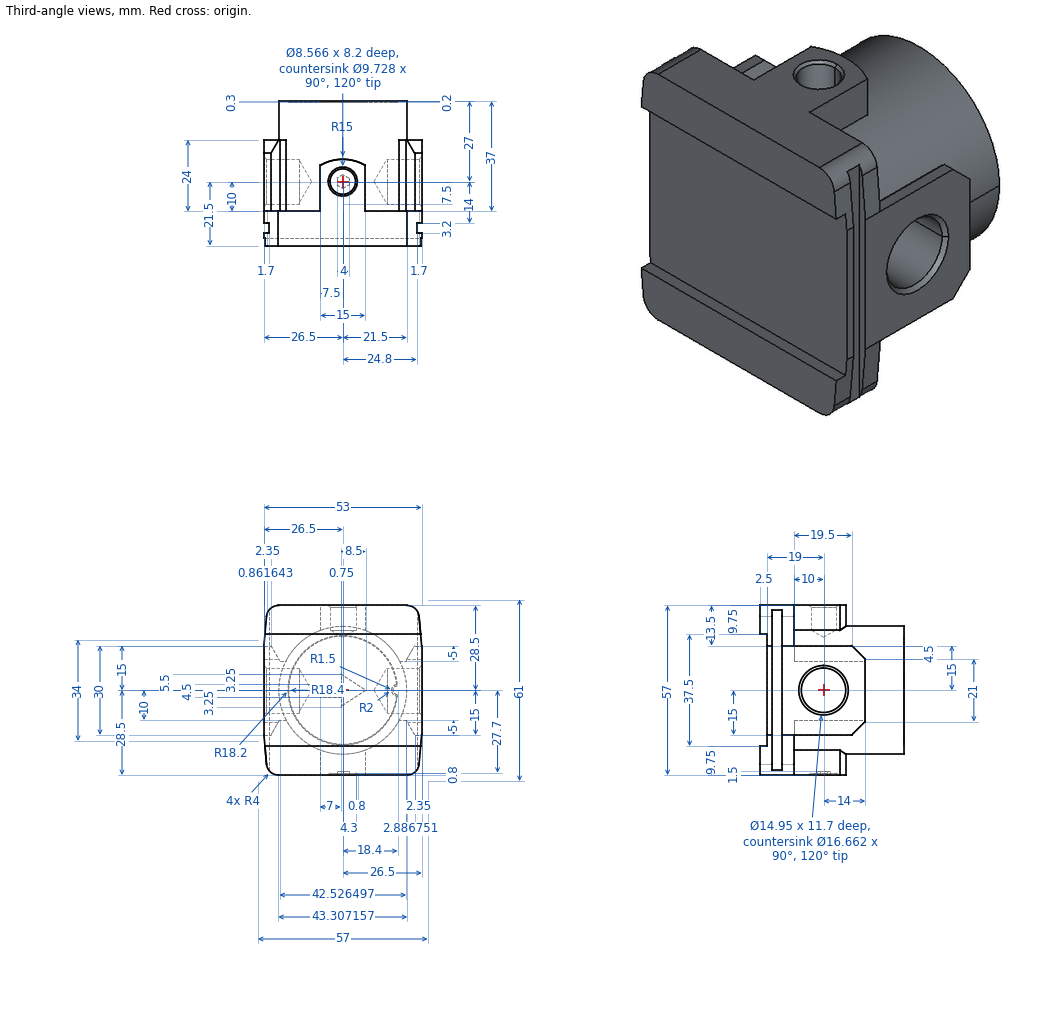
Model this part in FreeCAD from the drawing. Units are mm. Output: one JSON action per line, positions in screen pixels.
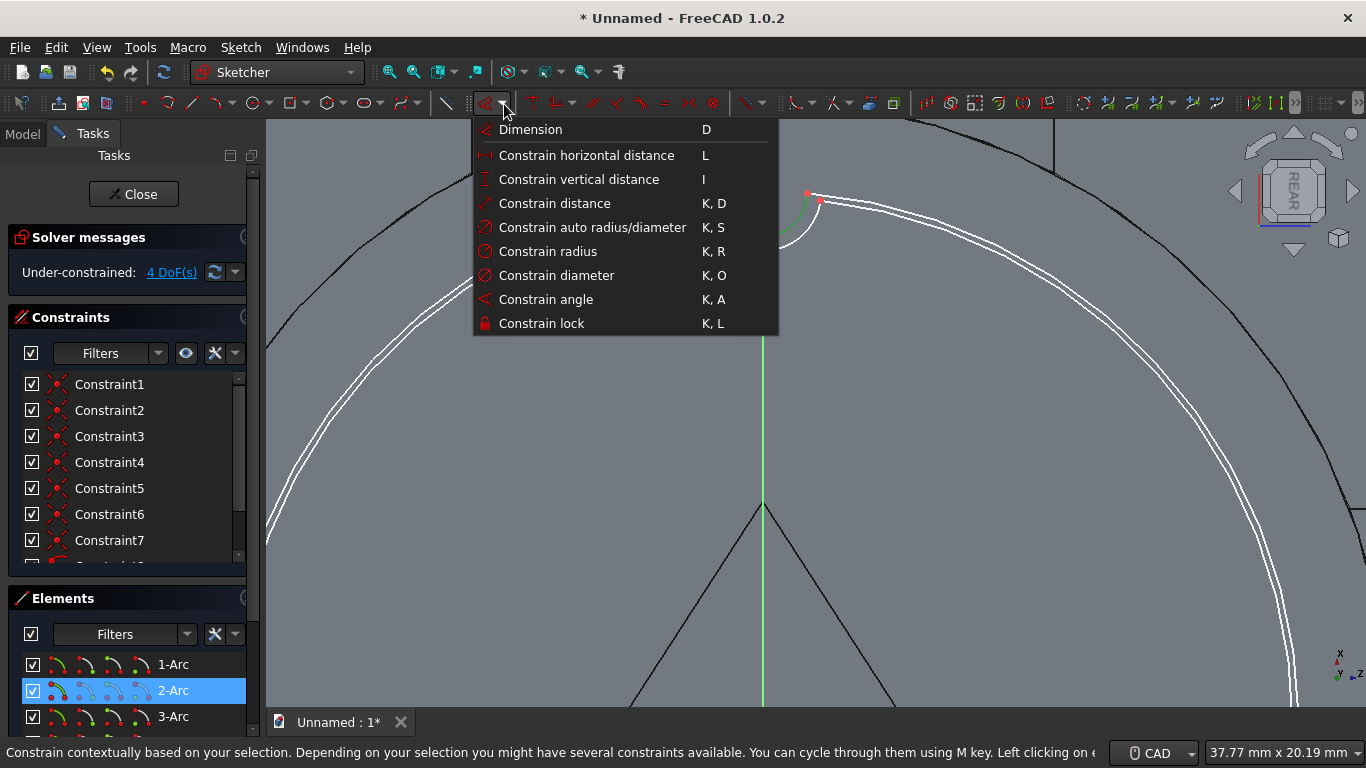
{"action": "left_click", "coordinate": [626, 251]}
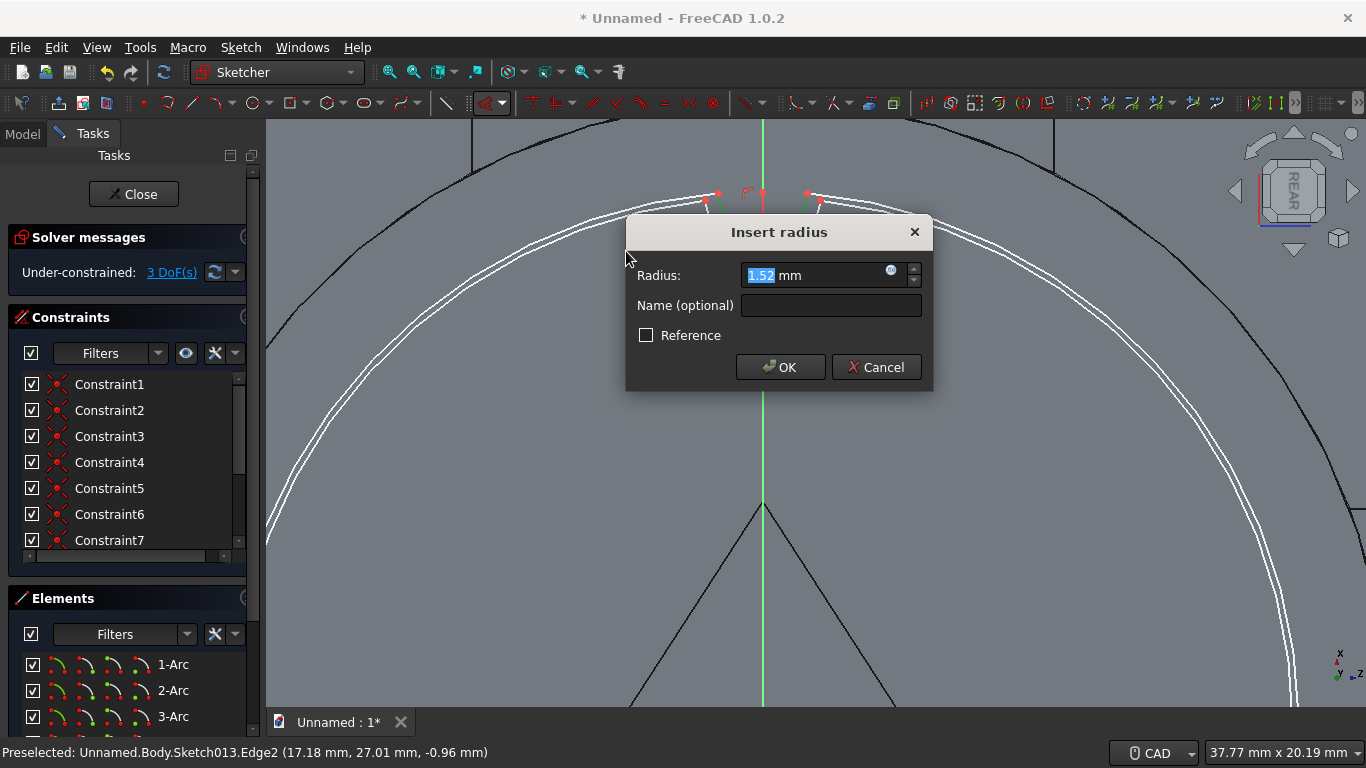
{"action": "type", "text": "1.5"}
{"action": "key", "text": "Return"}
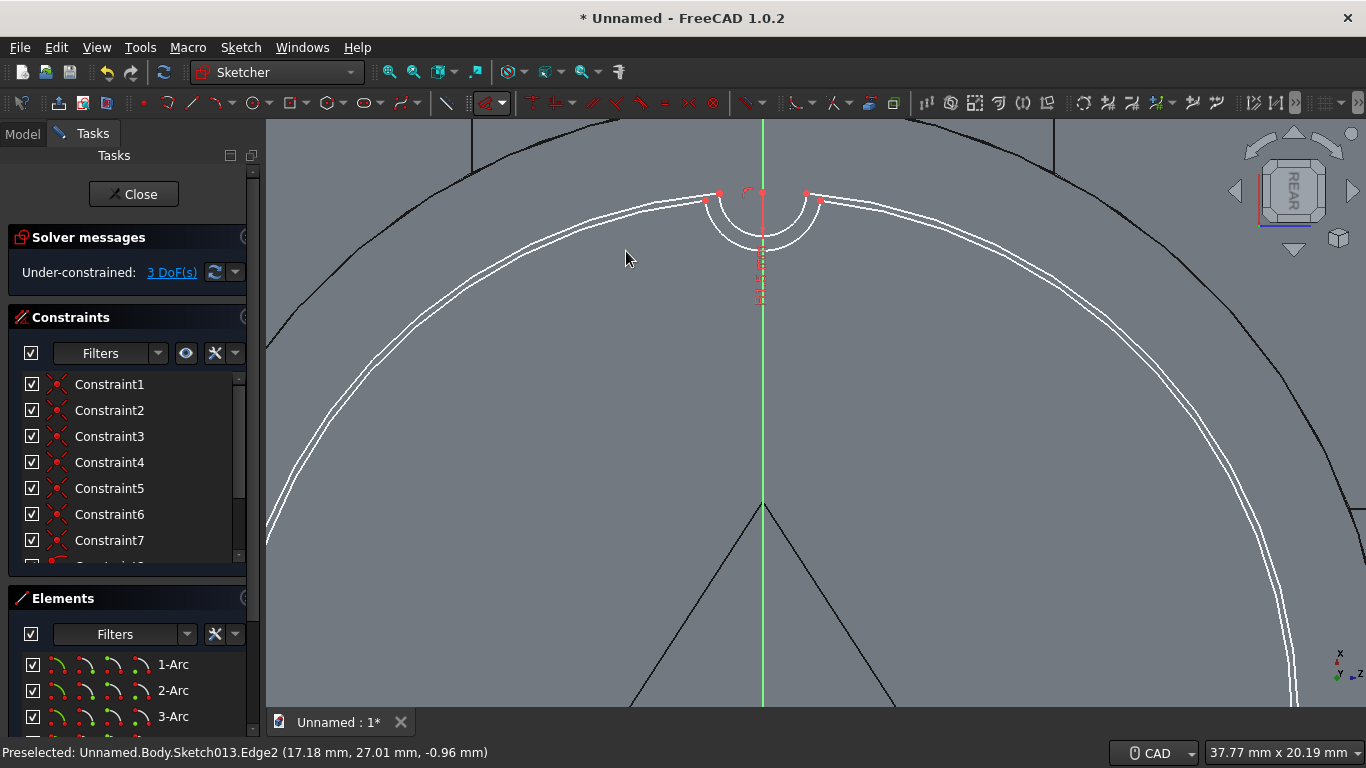
{"action": "scroll", "coordinate": [739, 230], "scroll_direction": "down", "scroll_amount": 5}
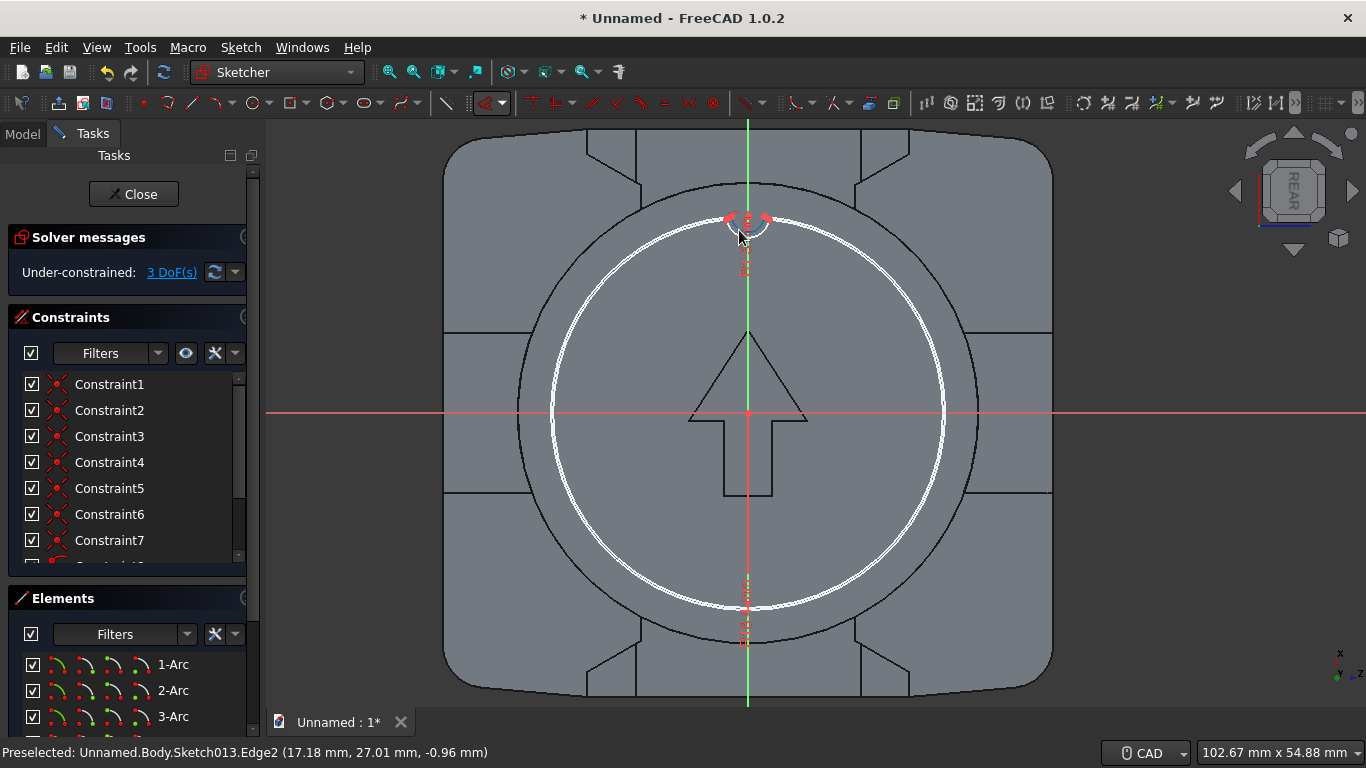
{"action": "scroll", "coordinate": [937, 365], "scroll_direction": "up", "scroll_amount": 10}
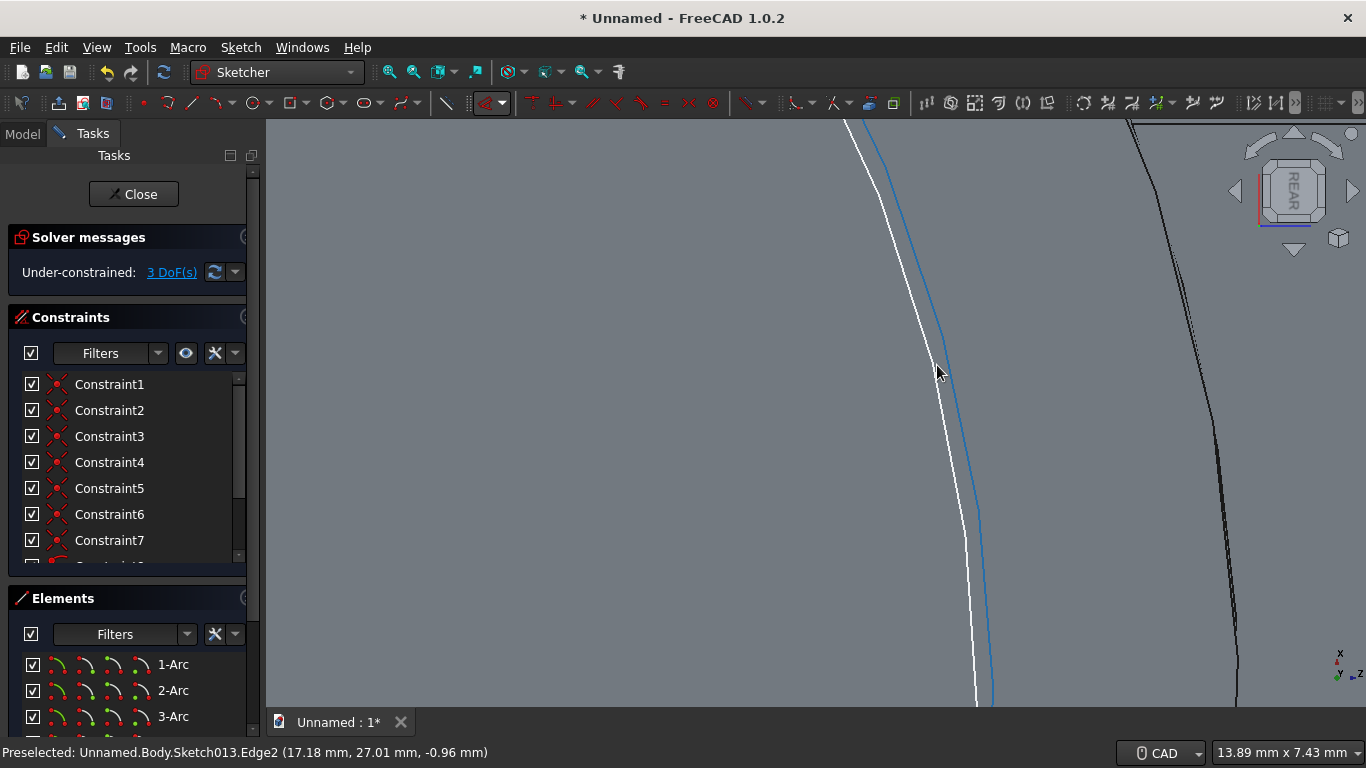
{"action": "left_click", "coordinate": [933, 363]}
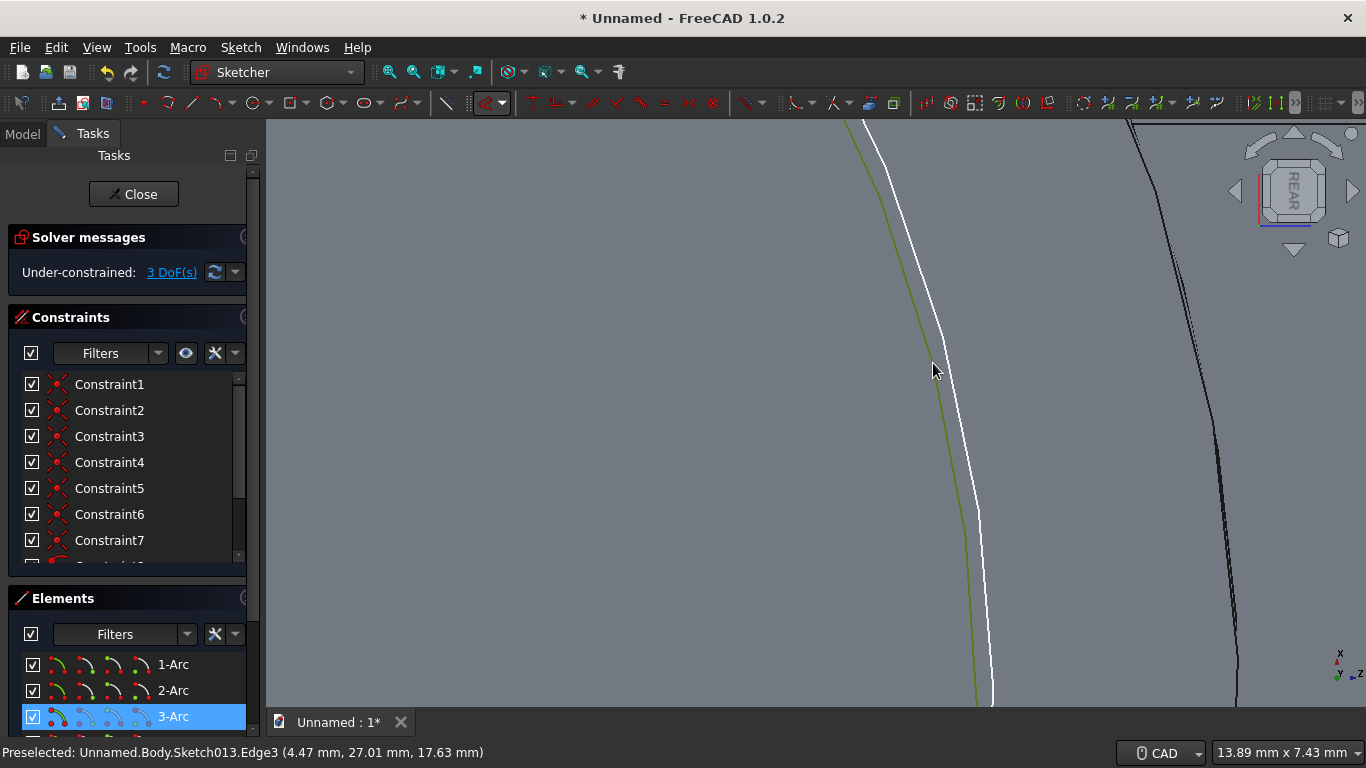
{"action": "key", "text": "k r"}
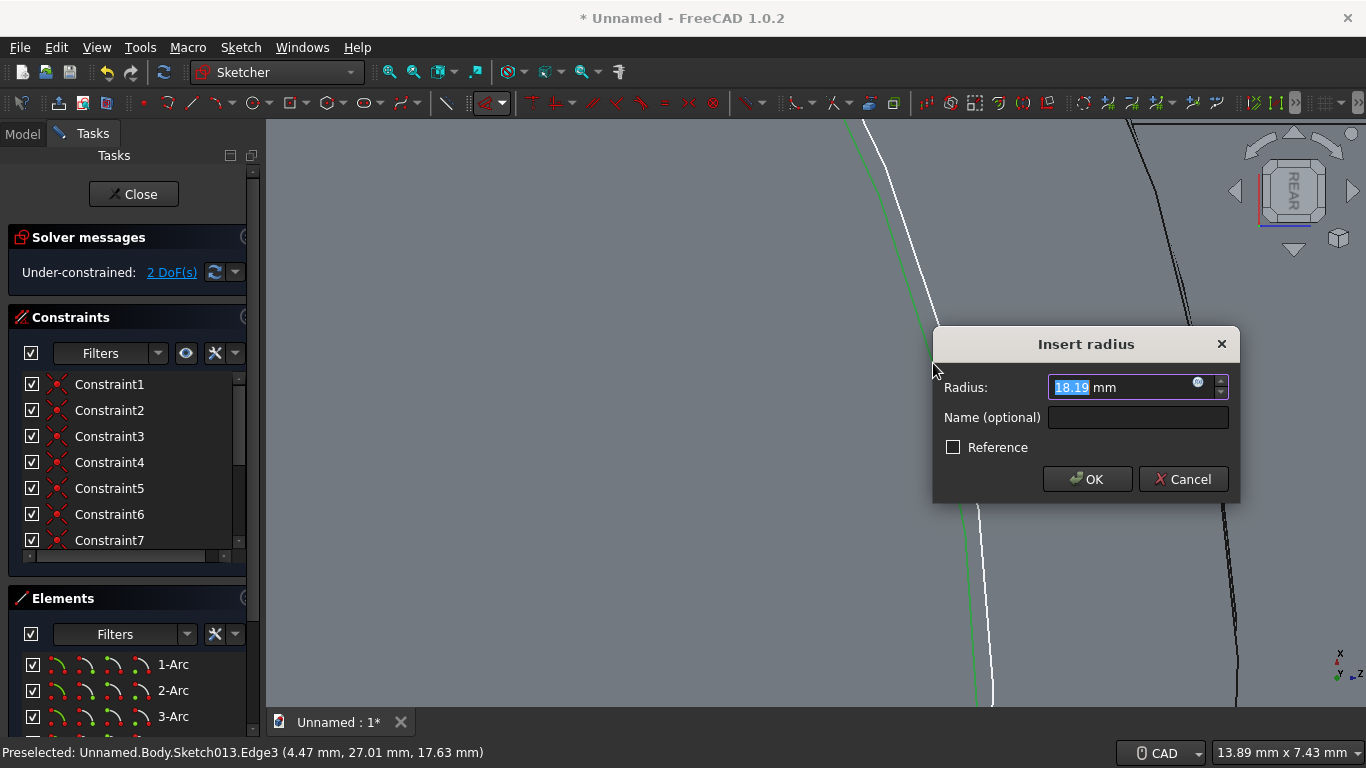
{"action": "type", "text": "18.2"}
{"action": "key", "text": "Return"}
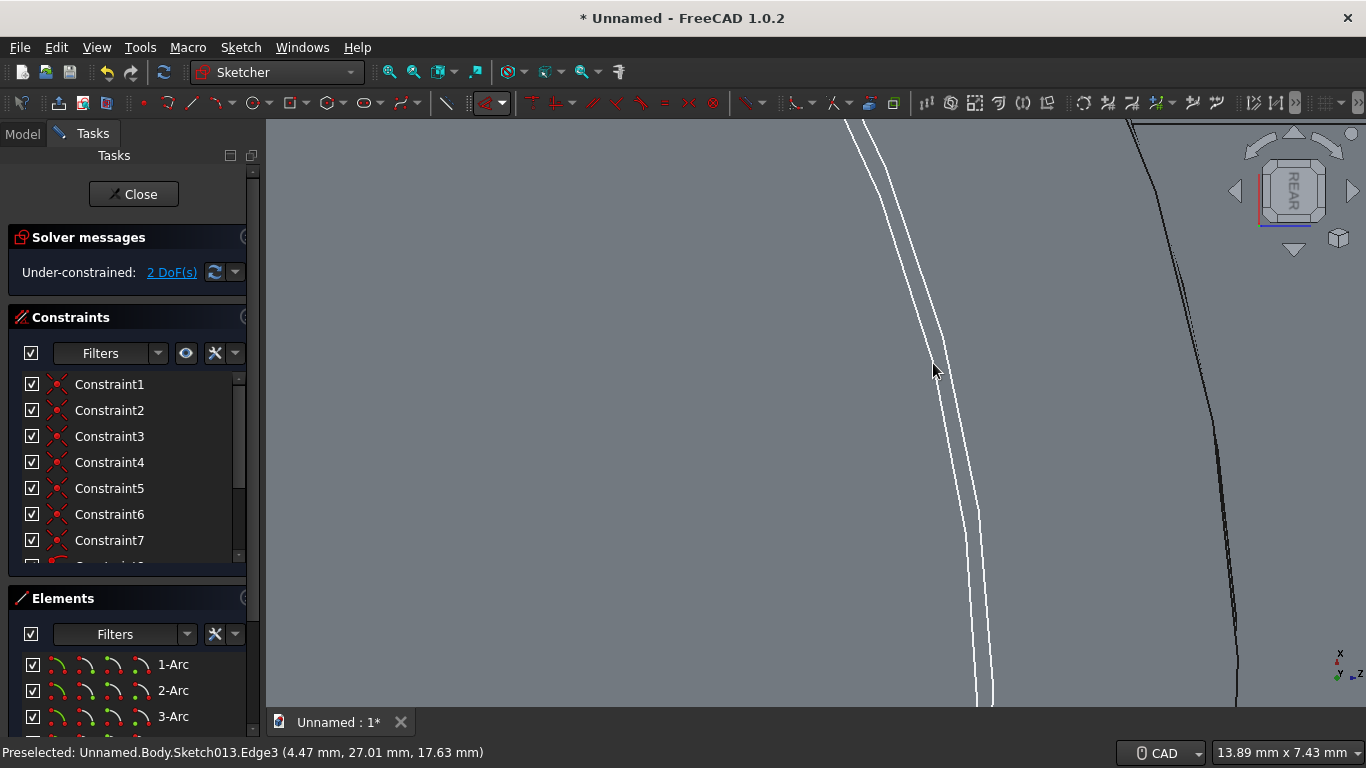
{"action": "scroll", "coordinate": [937, 365], "scroll_direction": "down", "scroll_amount": 10}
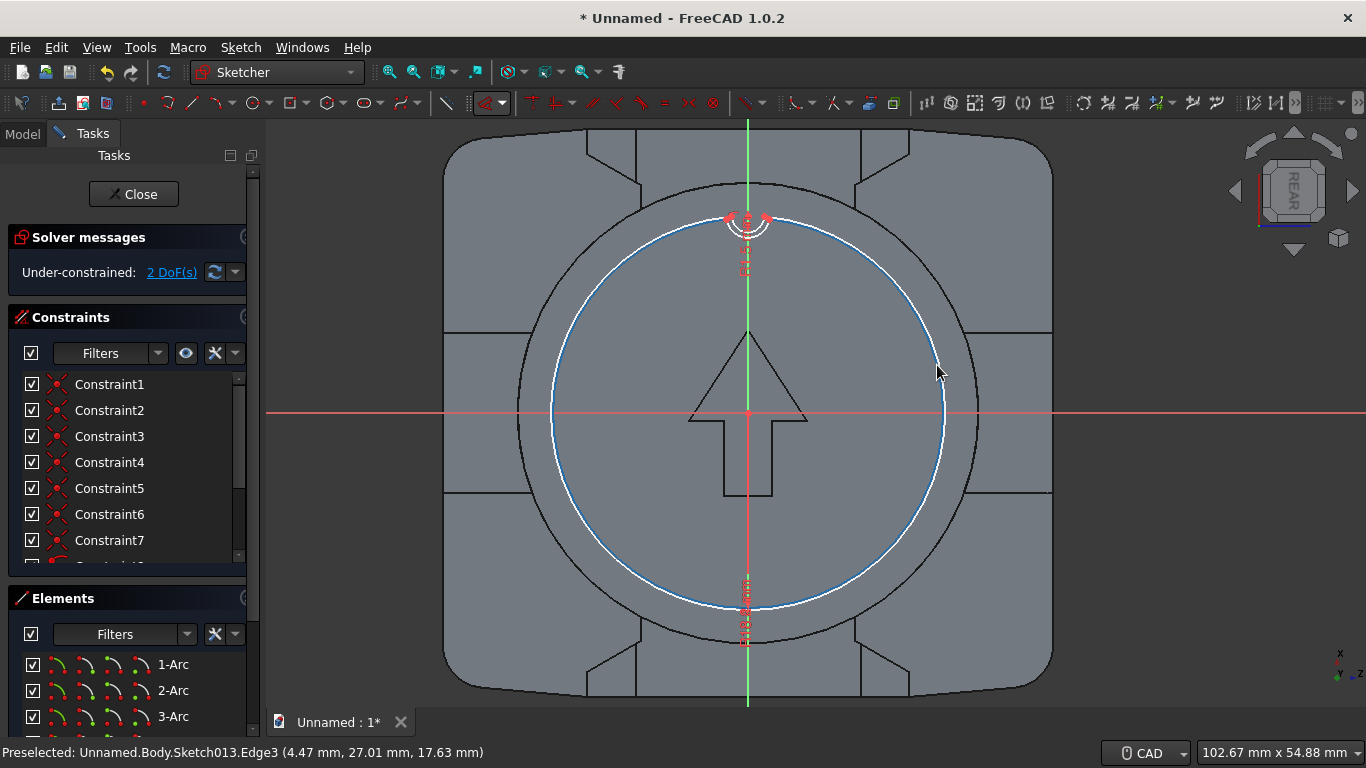
{"action": "scroll", "coordinate": [736, 234], "scroll_direction": "up", "scroll_amount": 5}